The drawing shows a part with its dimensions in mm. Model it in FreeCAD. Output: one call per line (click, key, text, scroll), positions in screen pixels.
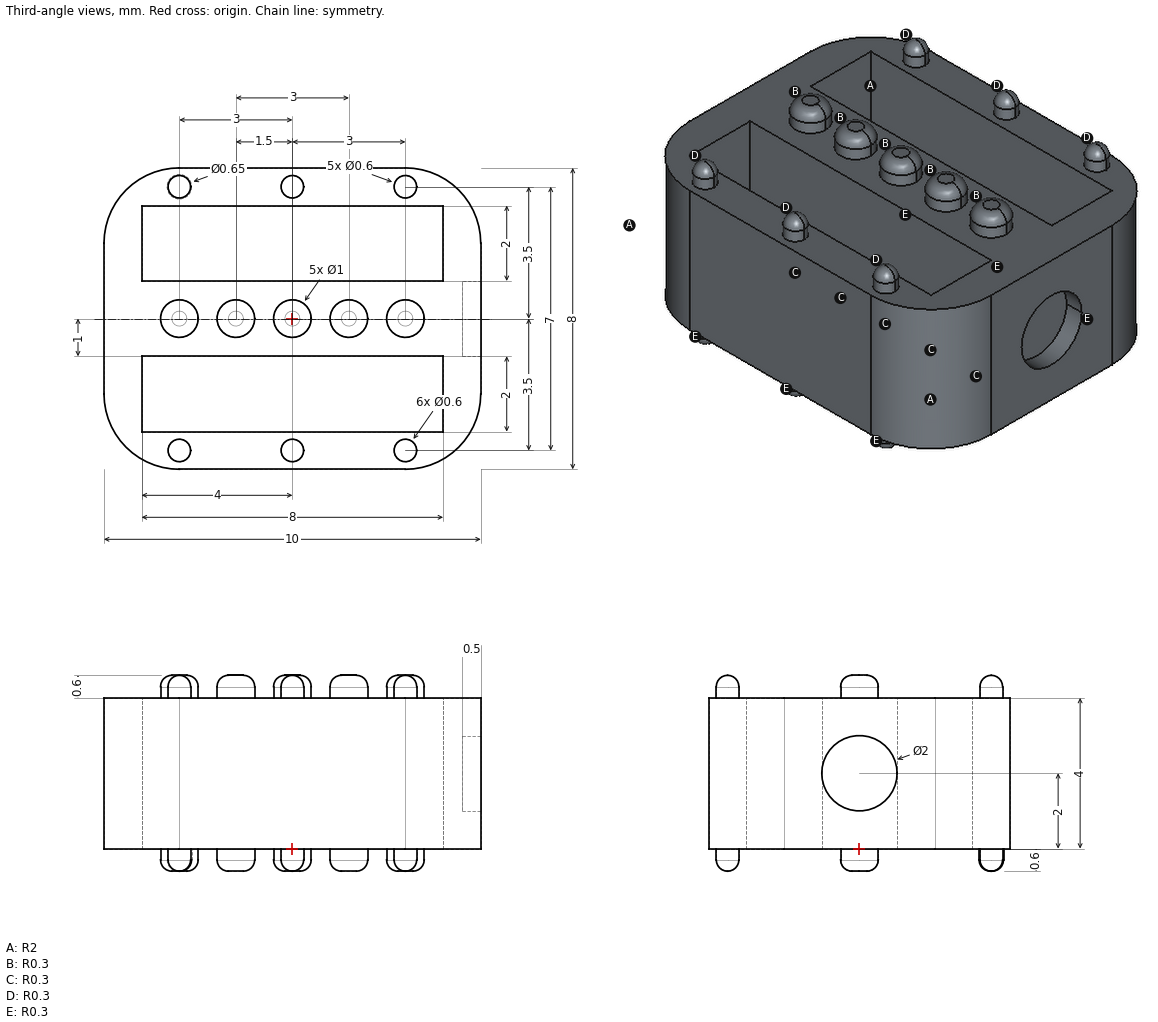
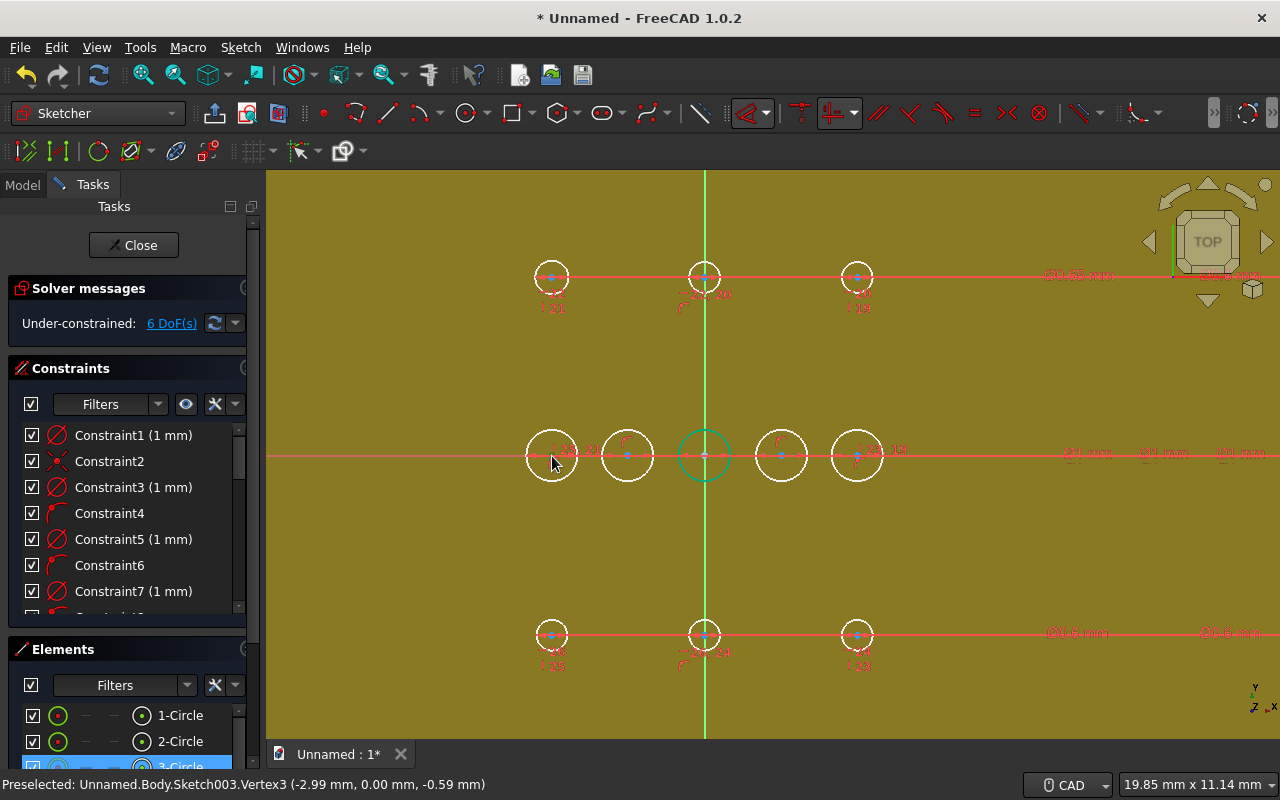
click(768, 114)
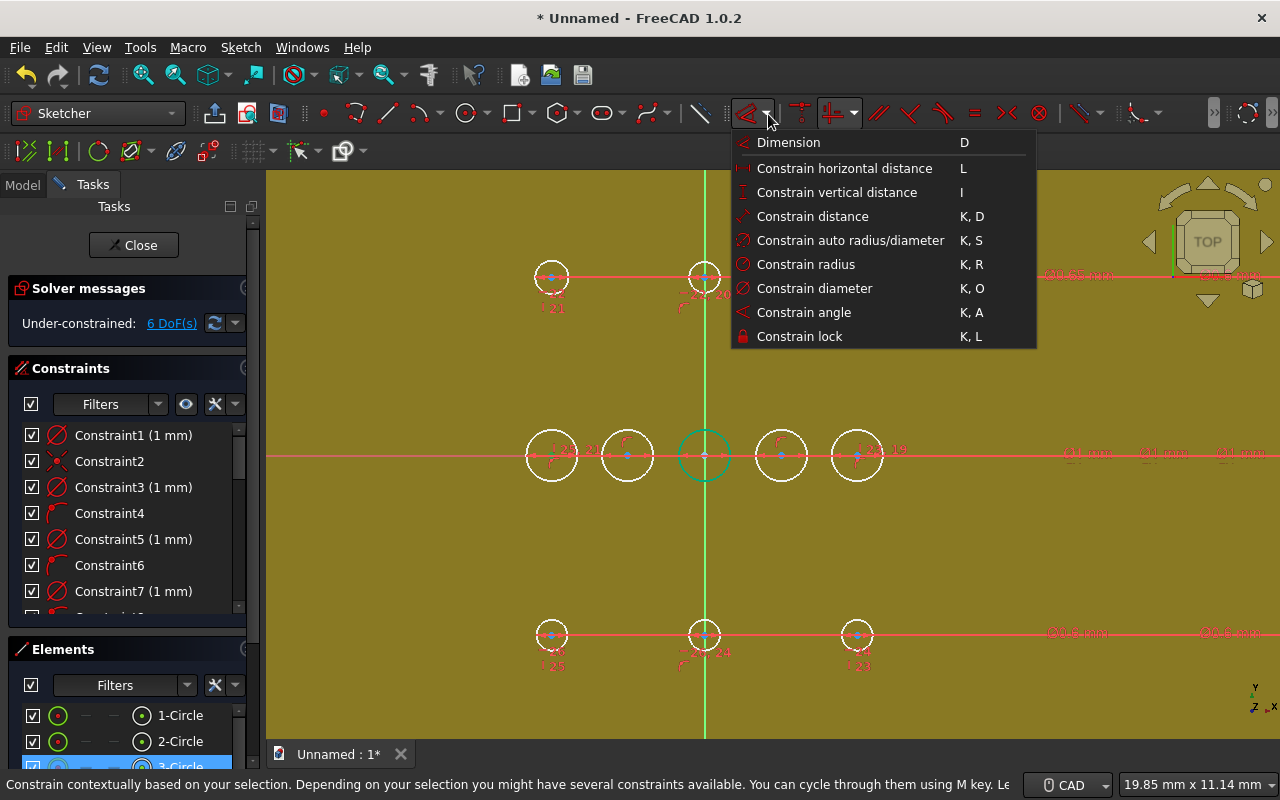
click(884, 168)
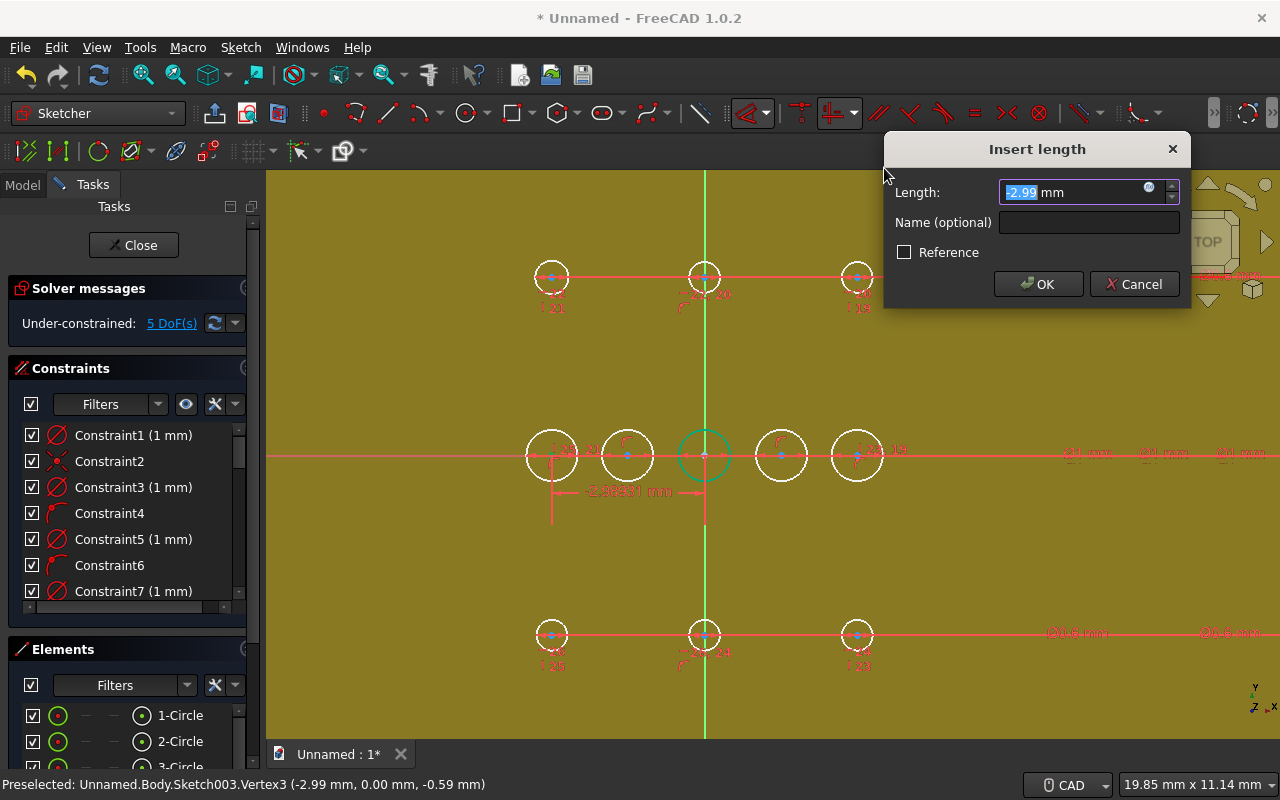
text(-3)
key(Return)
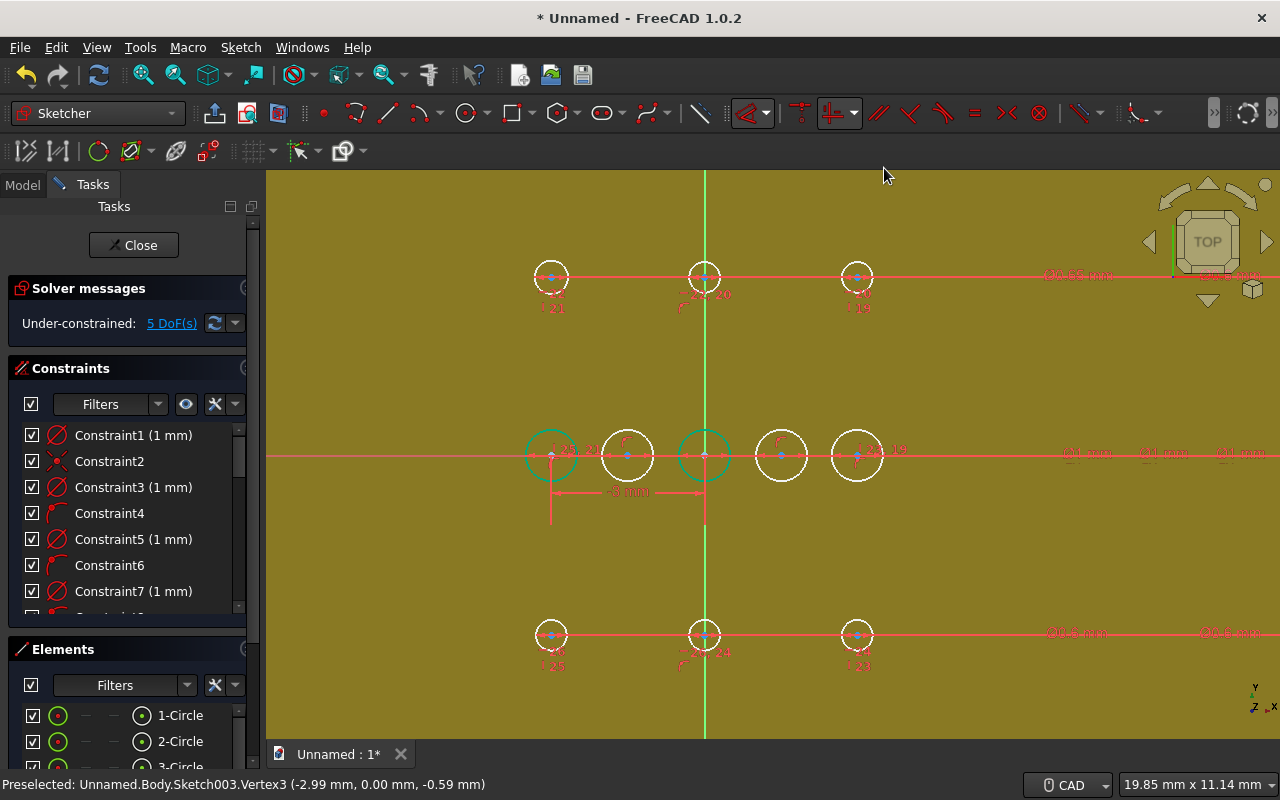
click(857, 456)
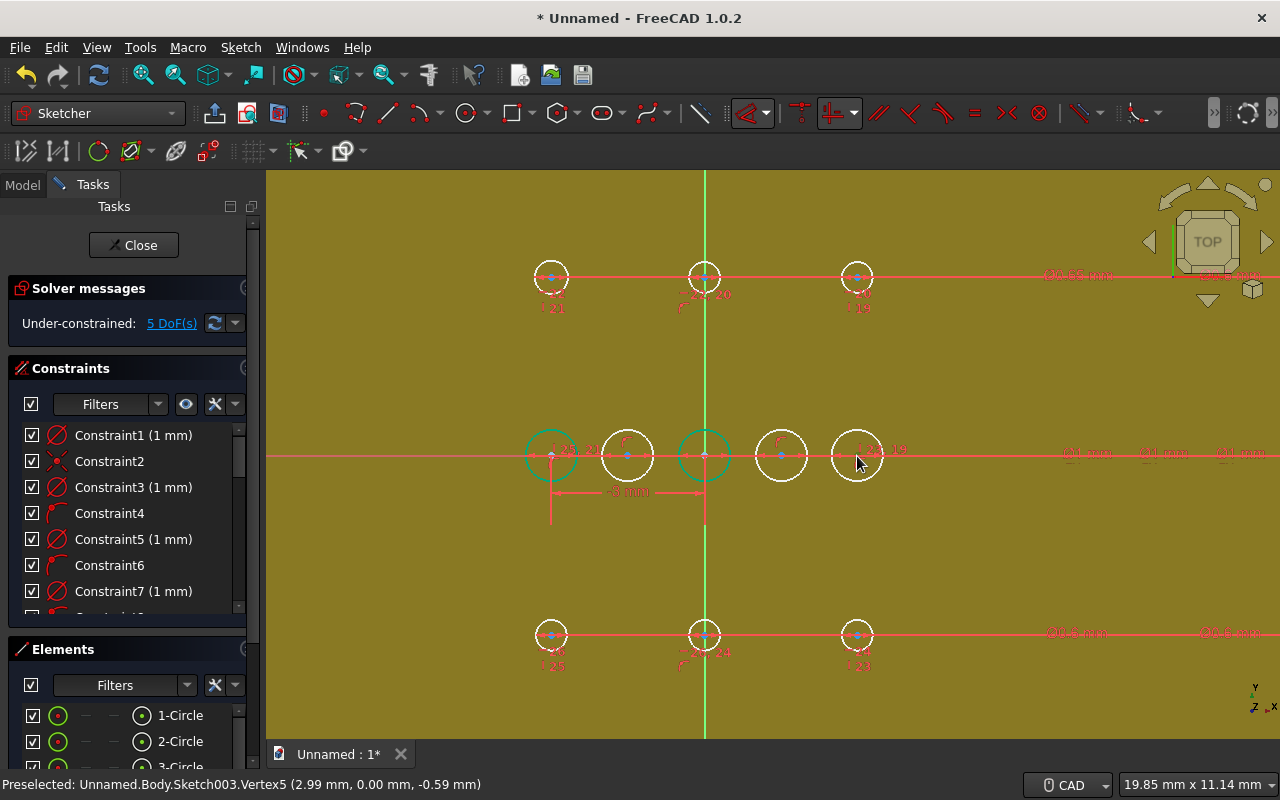
key(l)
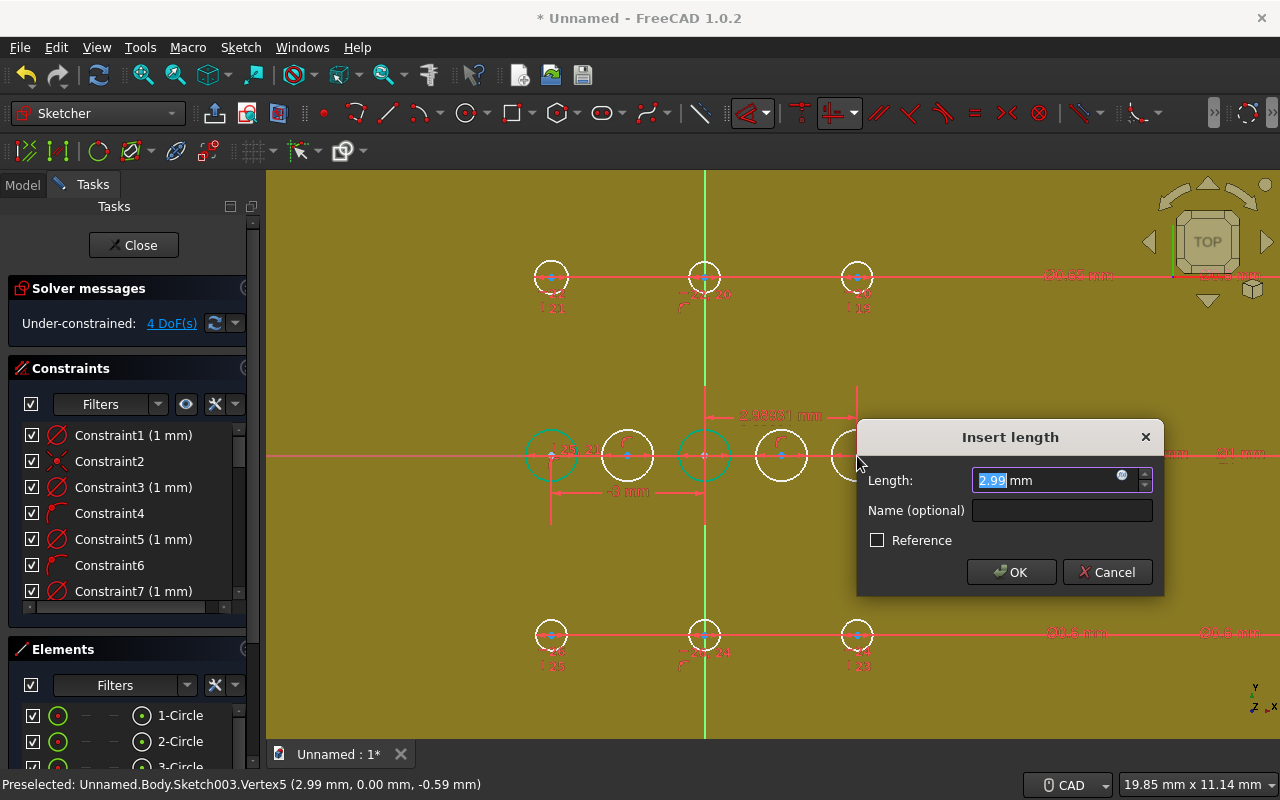
text(3)
key(Return)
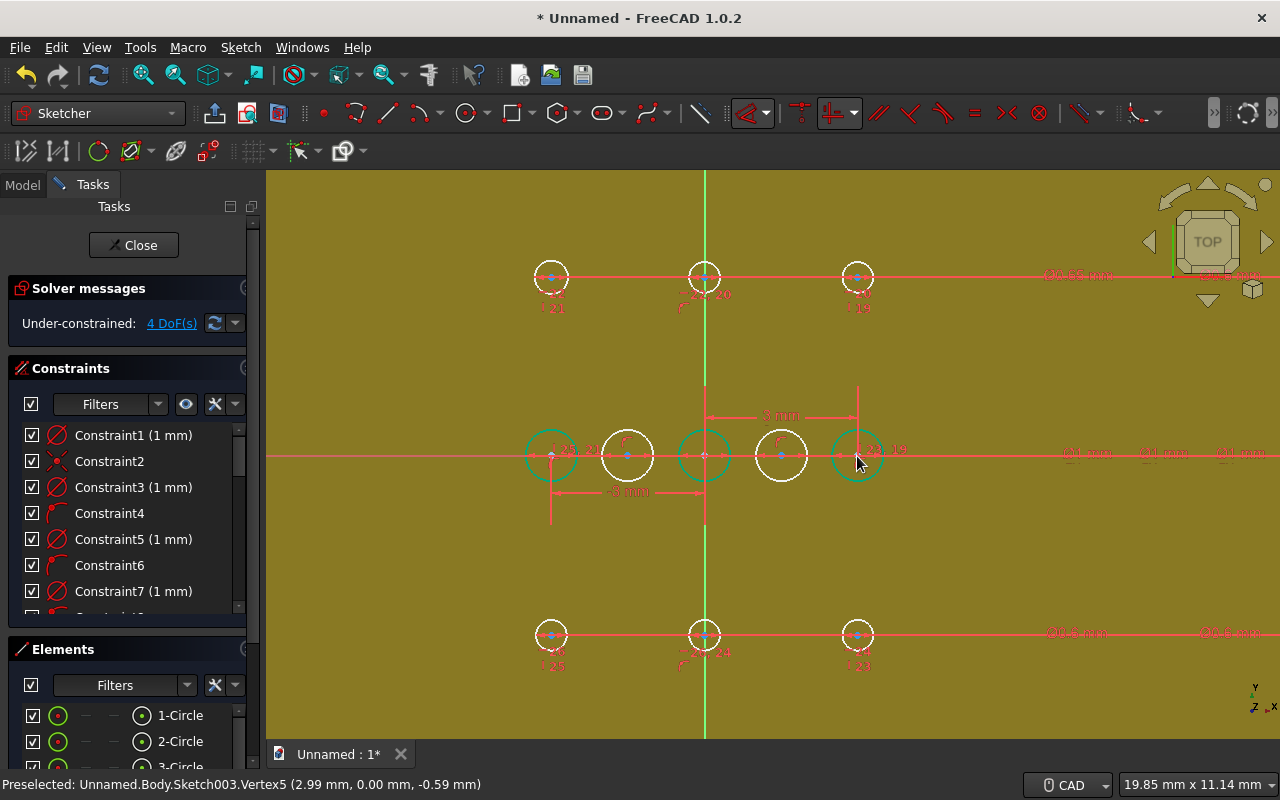
click(628, 456)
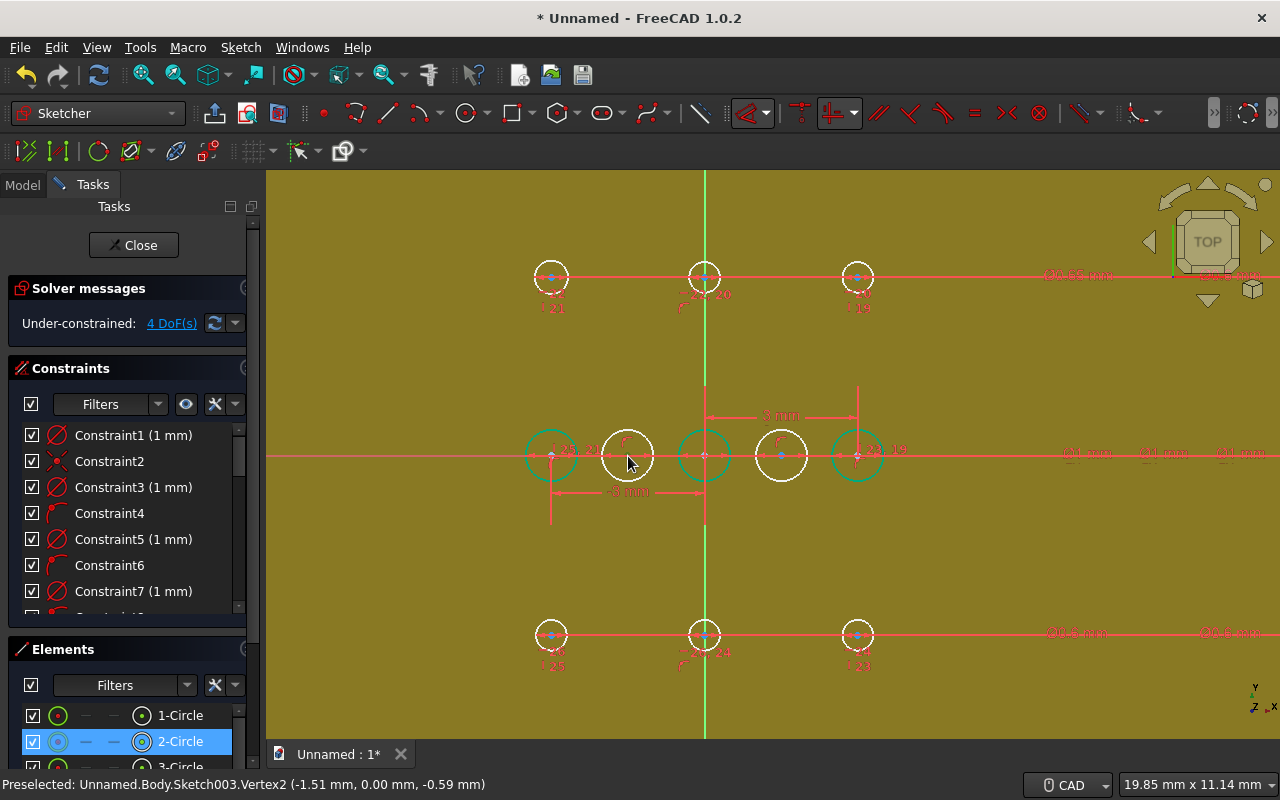
click(782, 456)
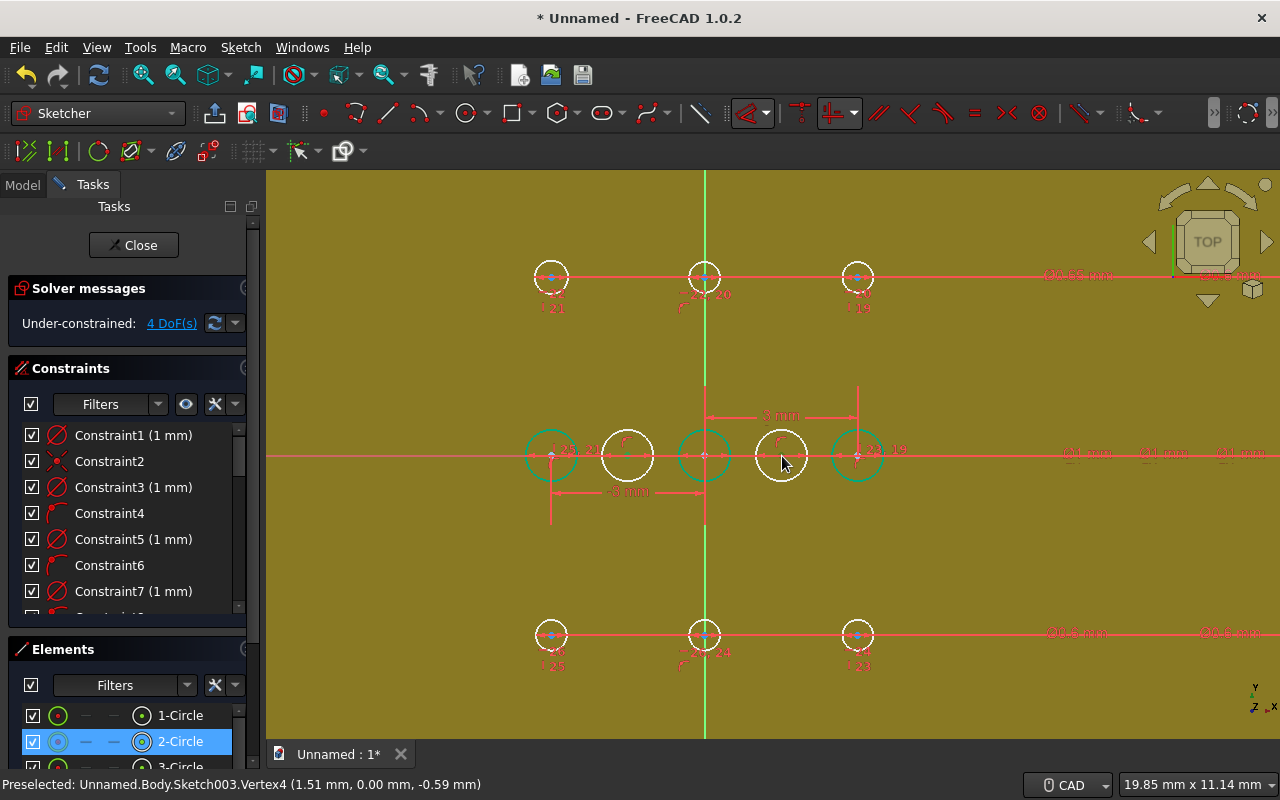
key(l)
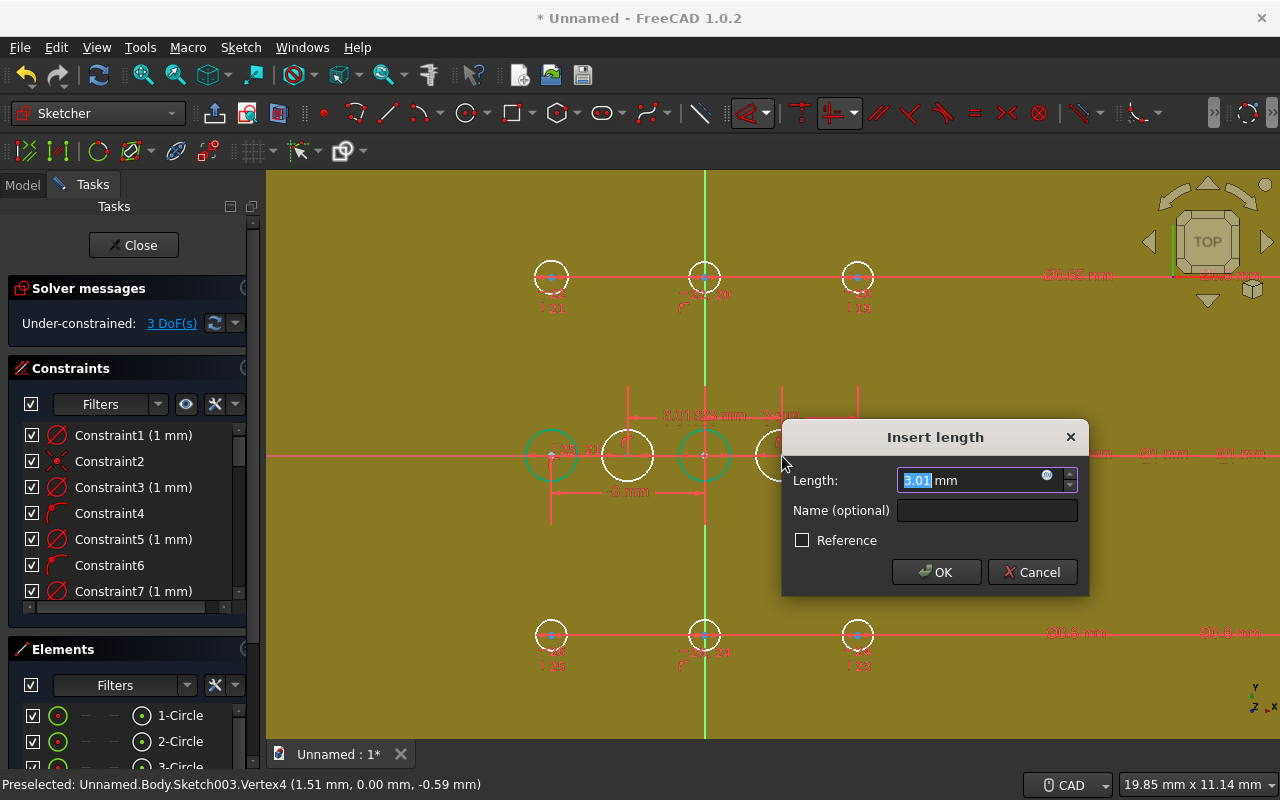
text(3)
key(Return)